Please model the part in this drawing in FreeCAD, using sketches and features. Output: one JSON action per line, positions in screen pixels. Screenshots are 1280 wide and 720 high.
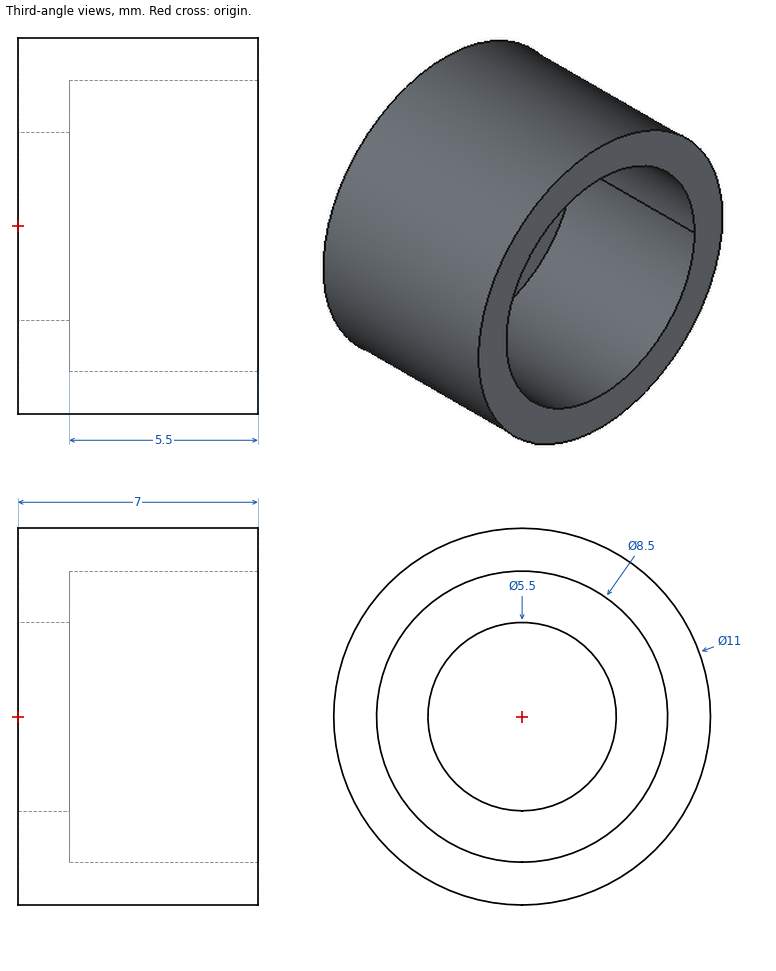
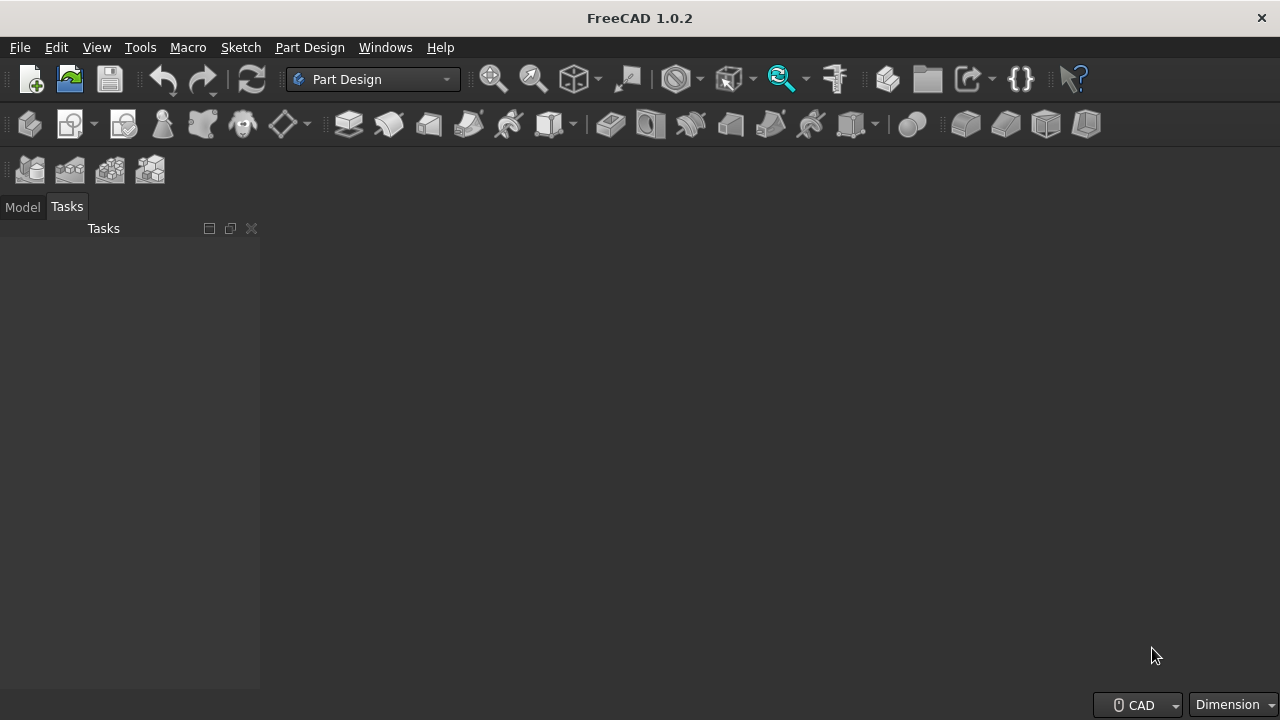
{"action": "left_click", "coordinate": [30, 80]}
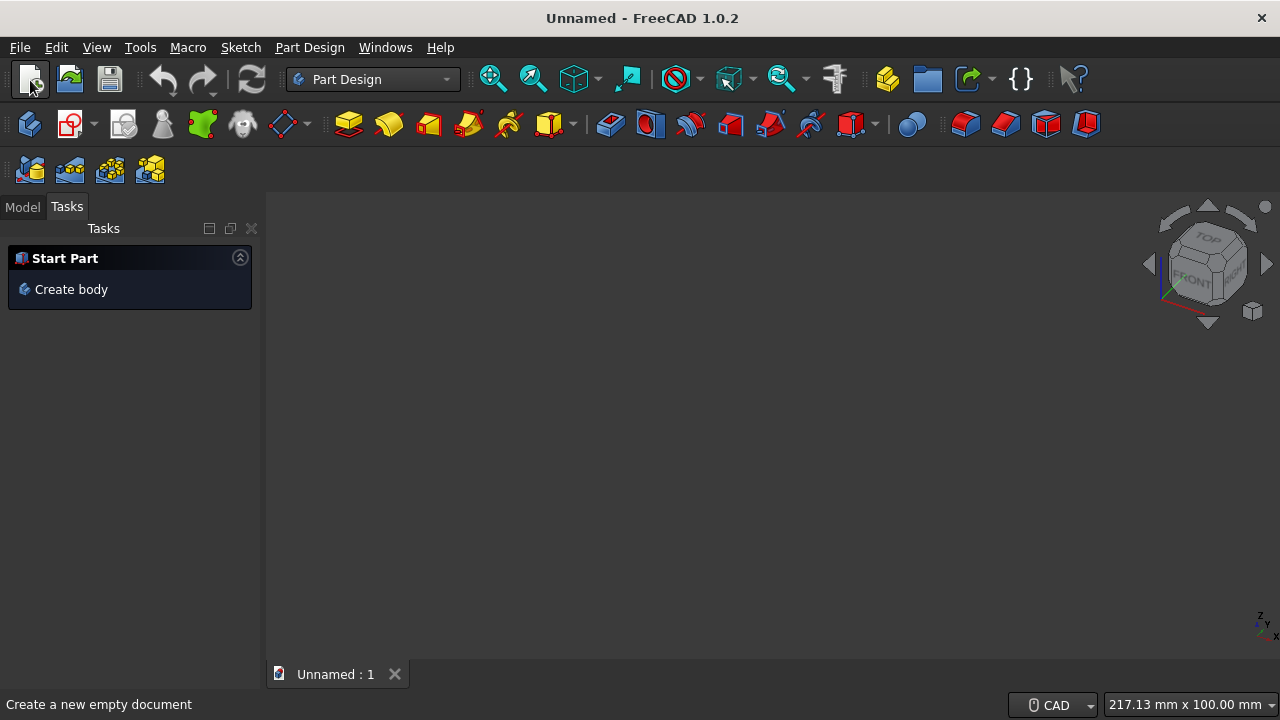
{"action": "left_click", "coordinate": [70, 124]}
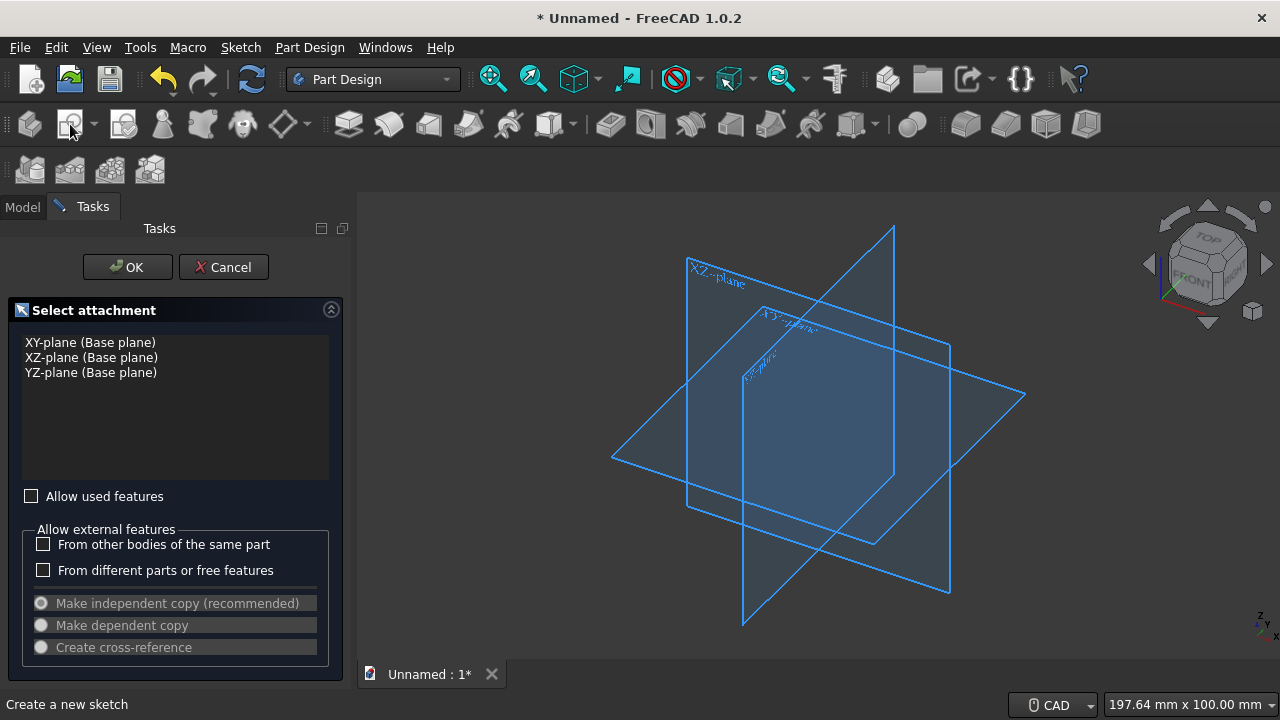
{"action": "left_click", "coordinate": [82, 372]}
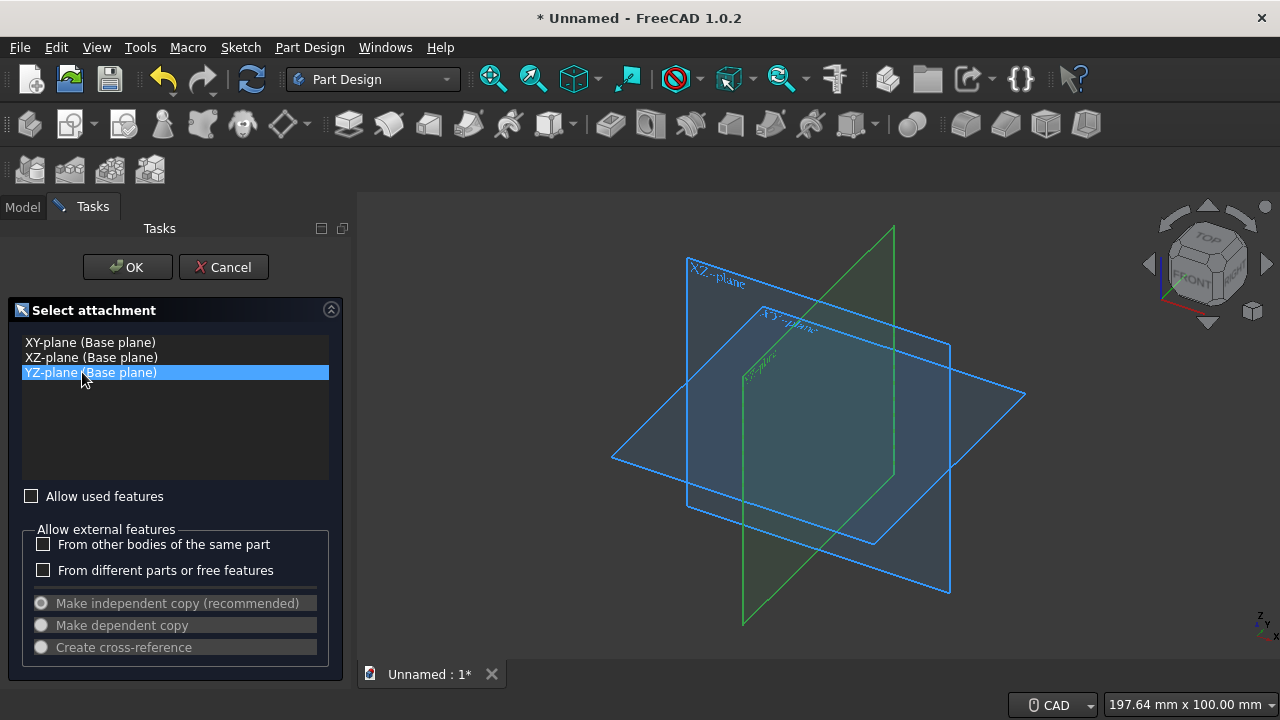
{"action": "left_click", "coordinate": [128, 267]}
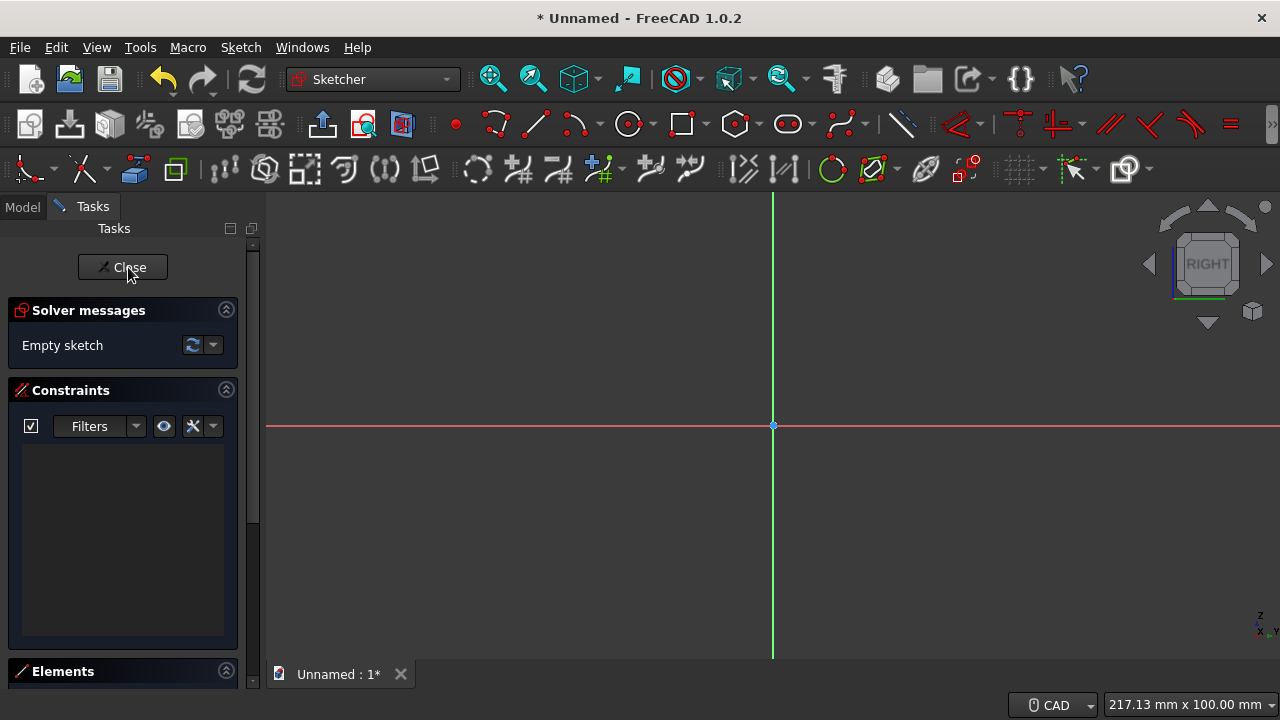
{"action": "scroll", "coordinate": [787, 426], "scroll_direction": "up", "scroll_amount": 9}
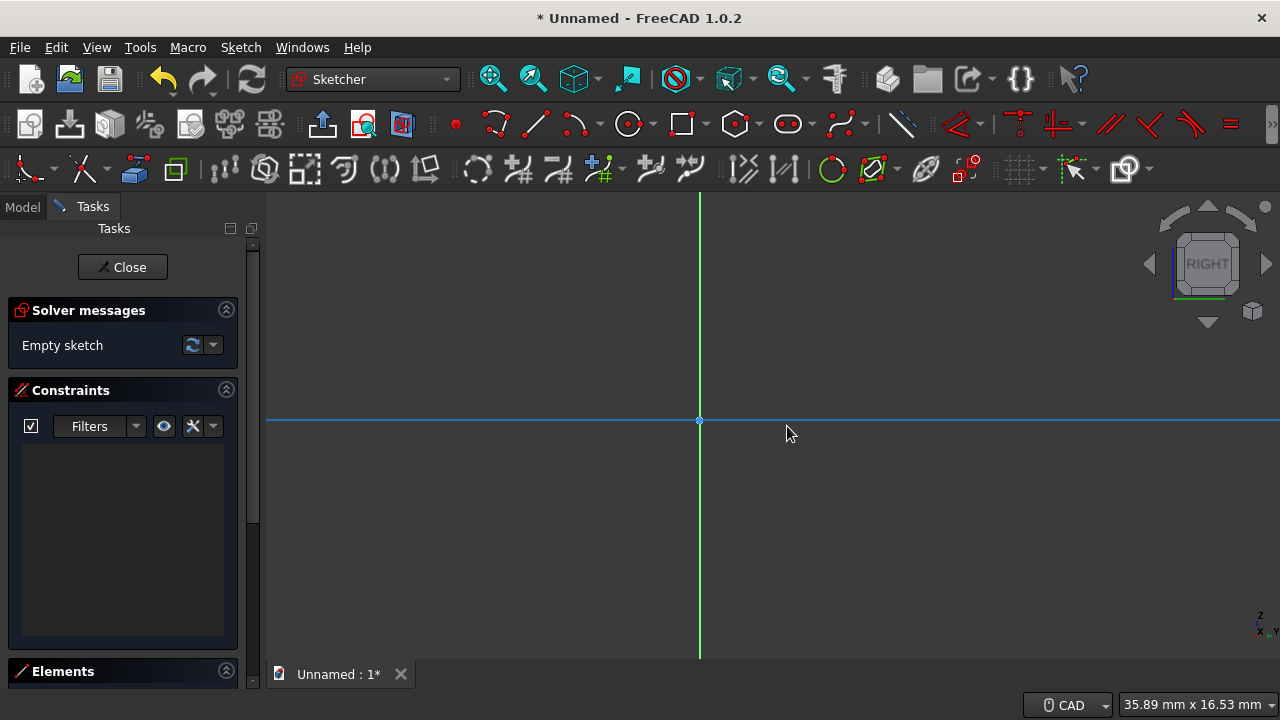
{"action": "left_click", "coordinate": [630, 124]}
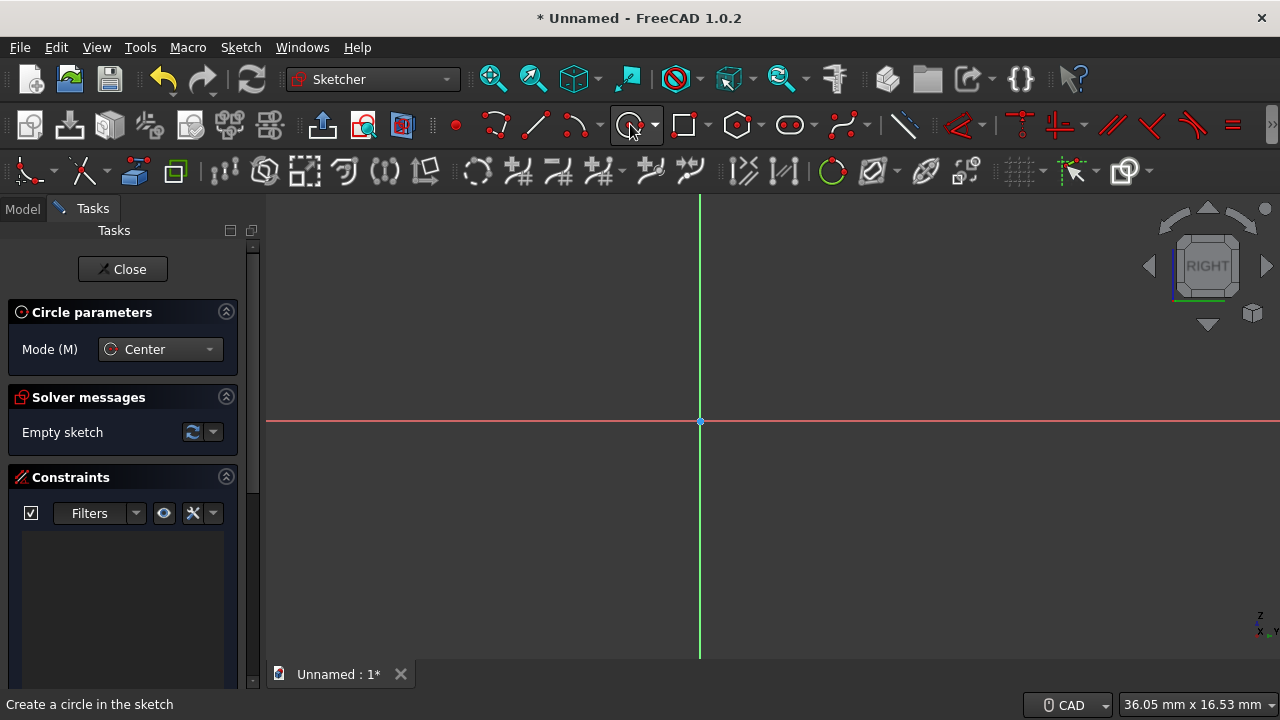
{"action": "left_click", "coordinate": [700, 421]}
{"action": "mouse_move", "coordinate": [809, 312]}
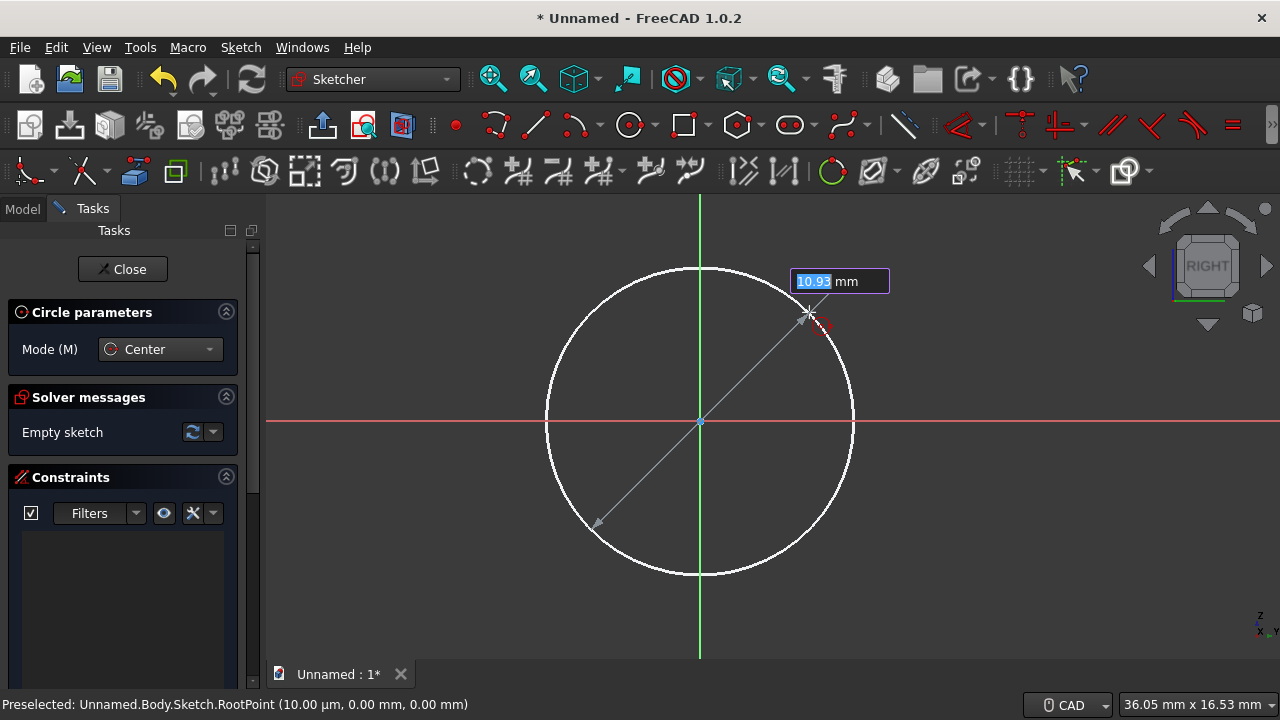
{"action": "type", "text": "11"}
{"action": "key", "text": "Return"}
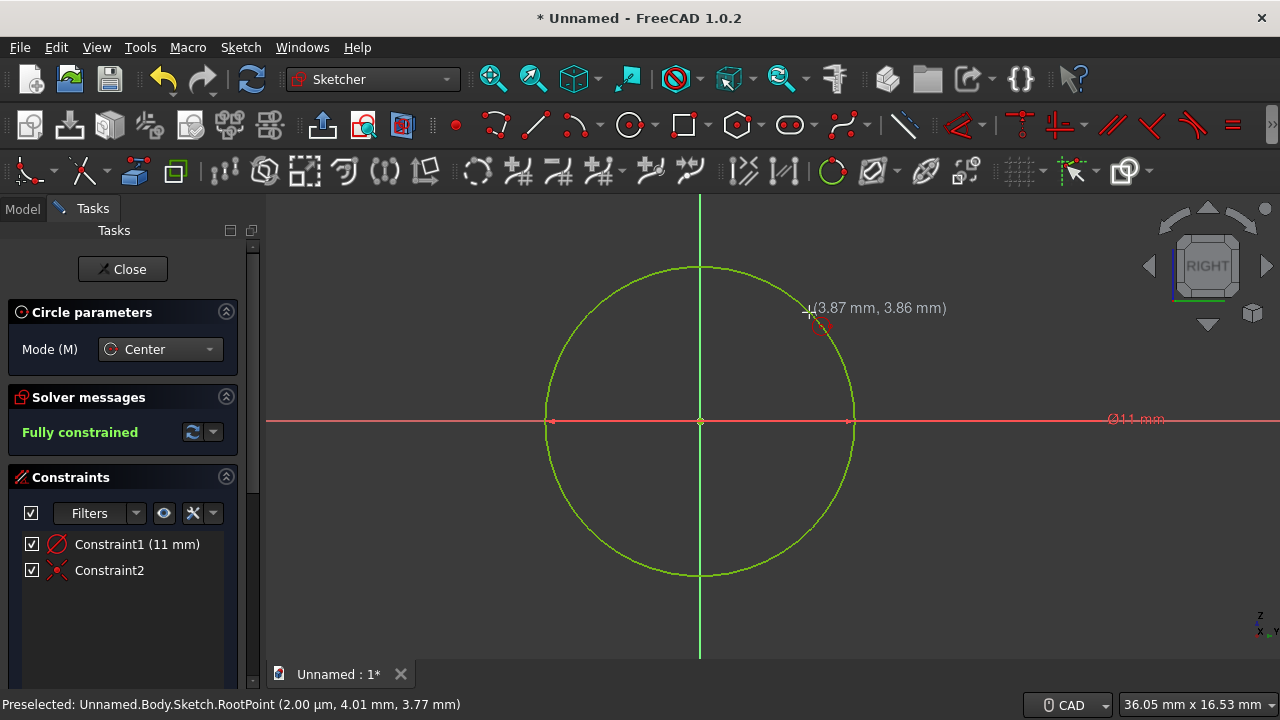
{"action": "left_click", "coordinate": [700, 421]}
{"action": "mouse_move", "coordinate": [755, 367]}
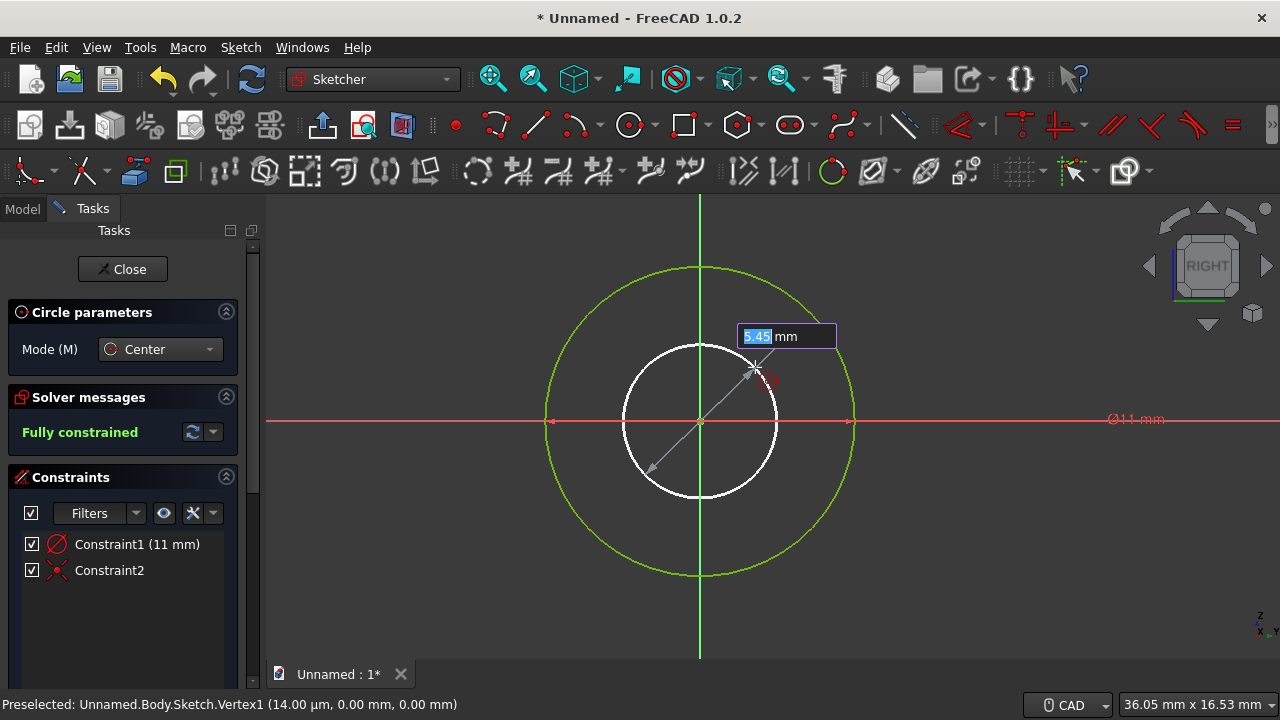
{"action": "type", "text": "5.5"}
{"action": "key", "text": "Return"}
{"action": "key", "text": "Escape"}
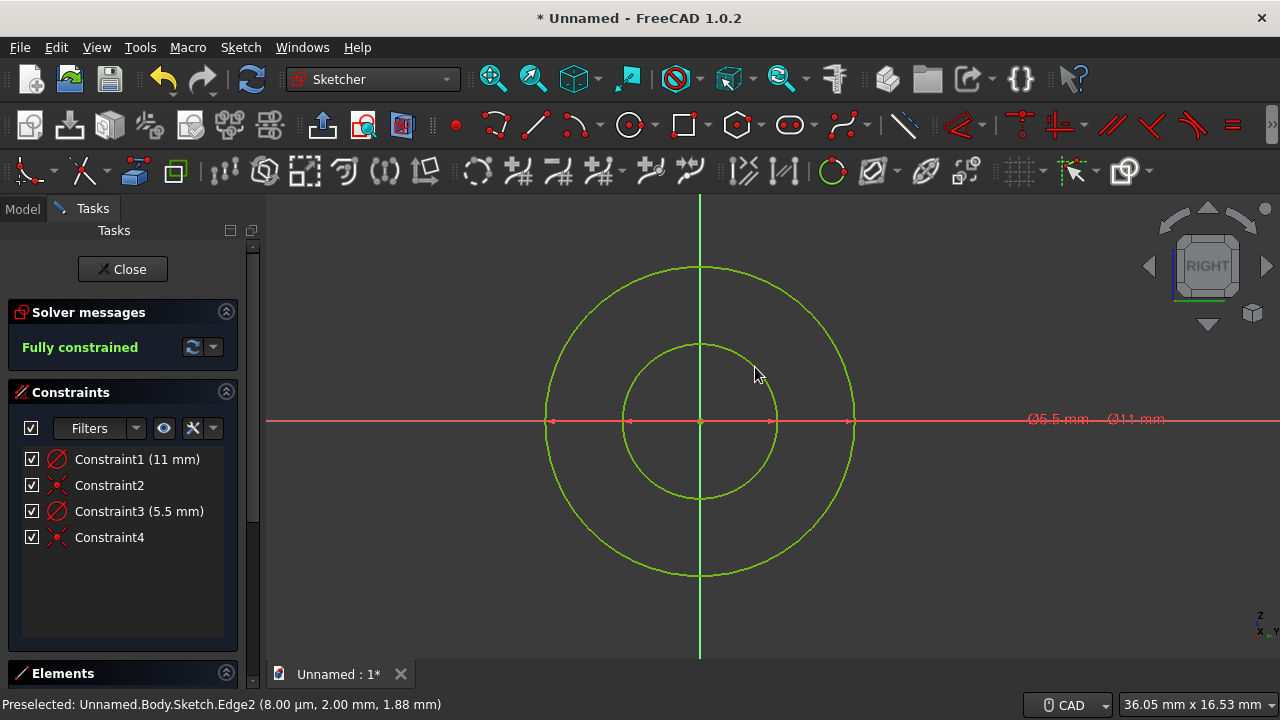
{"action": "left_click", "coordinate": [123, 269]}